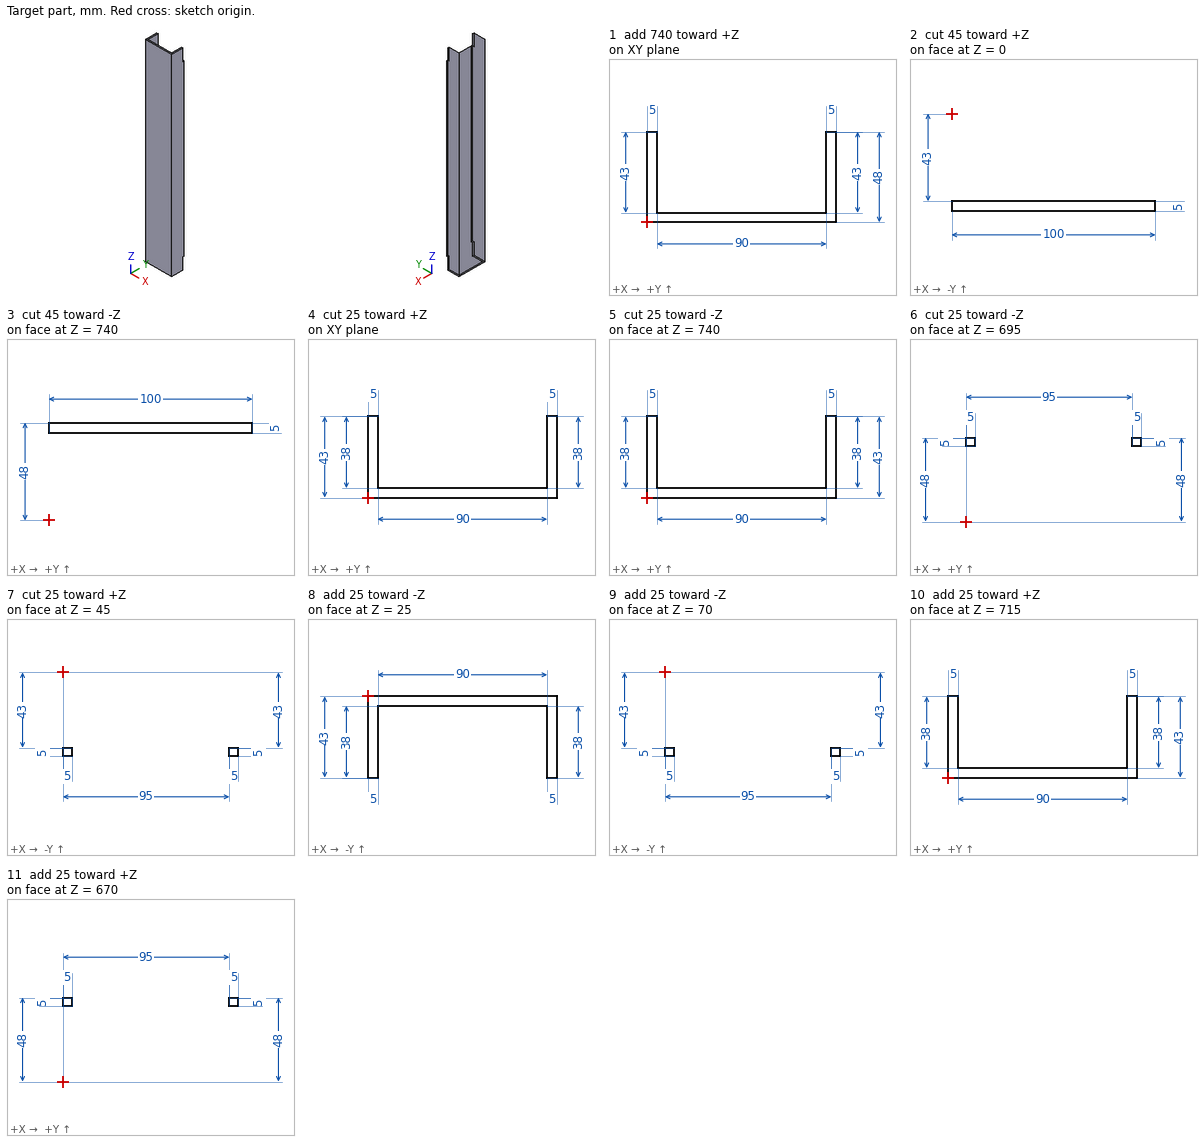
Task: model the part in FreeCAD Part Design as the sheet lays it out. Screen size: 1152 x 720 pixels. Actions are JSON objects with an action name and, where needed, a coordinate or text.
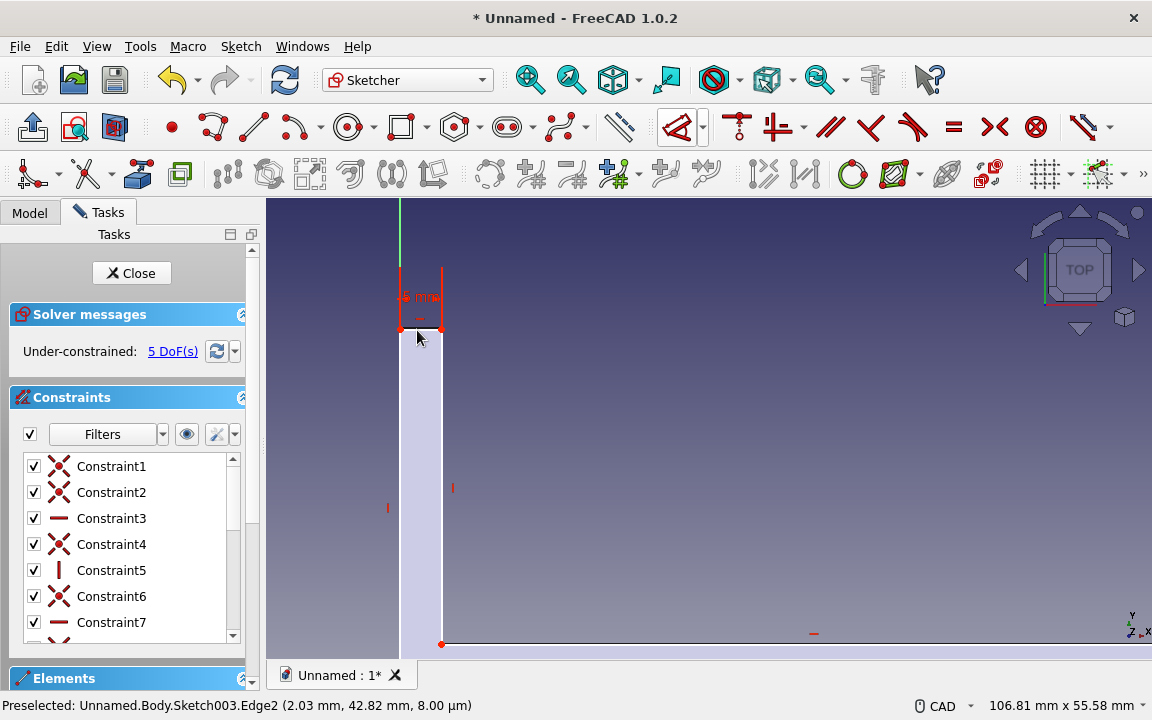
{"action": "scroll", "coordinate": [428, 333], "scroll_direction": "down", "scroll_amount": 3}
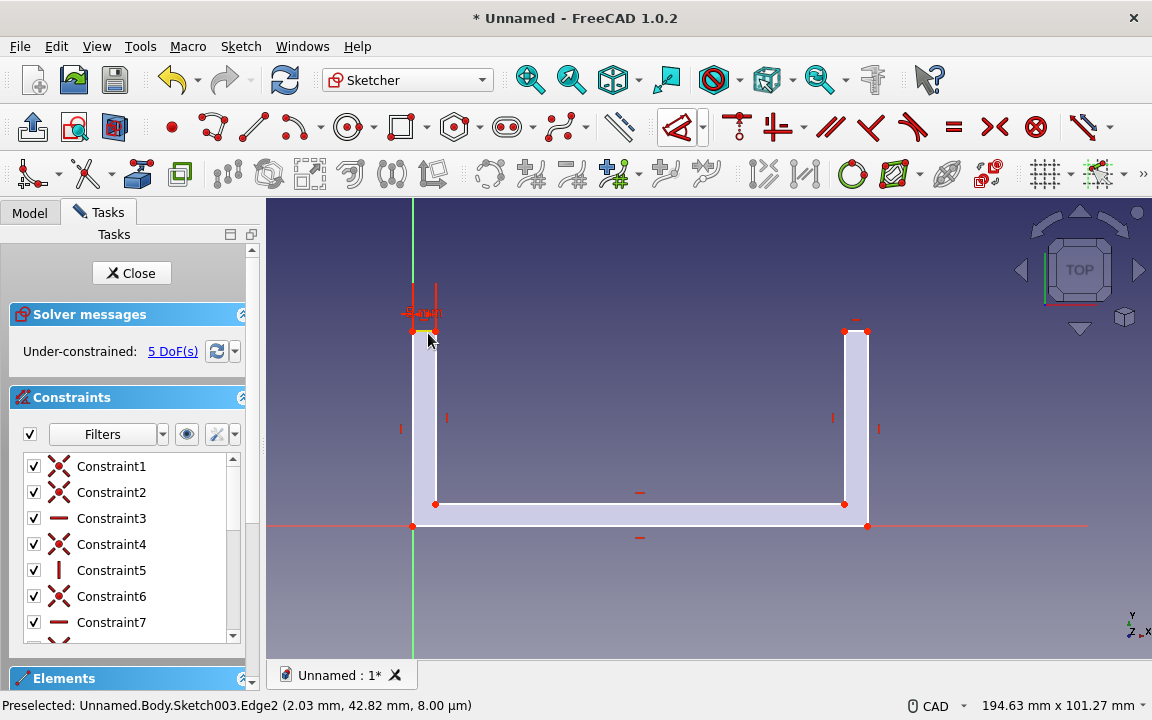
{"action": "scroll", "coordinate": [852, 331], "scroll_direction": "up", "scroll_amount": 4}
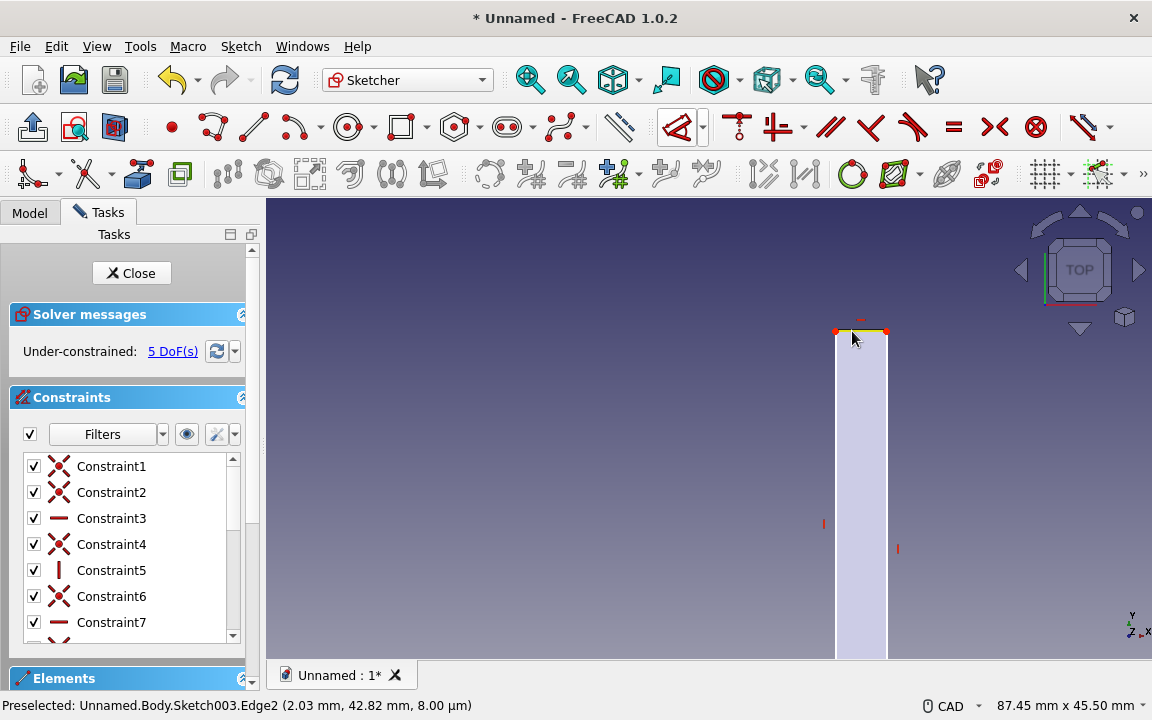
{"action": "left_click", "coordinate": [851, 331]}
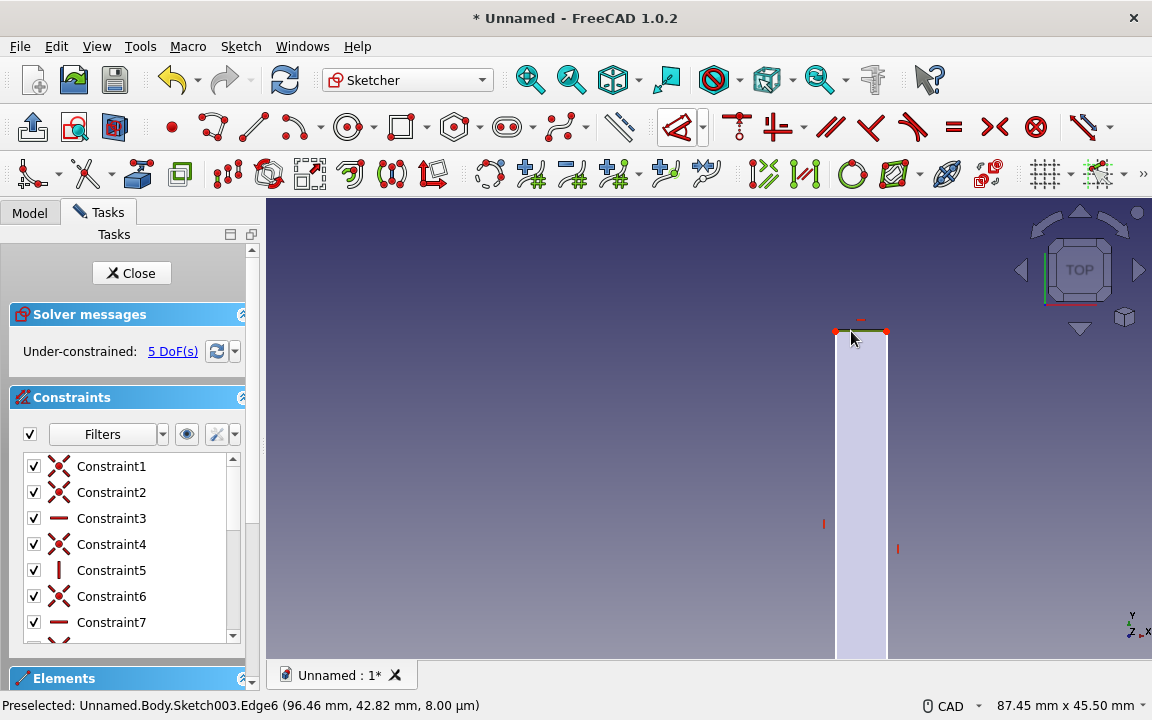
{"action": "left_click", "coordinate": [702, 128]}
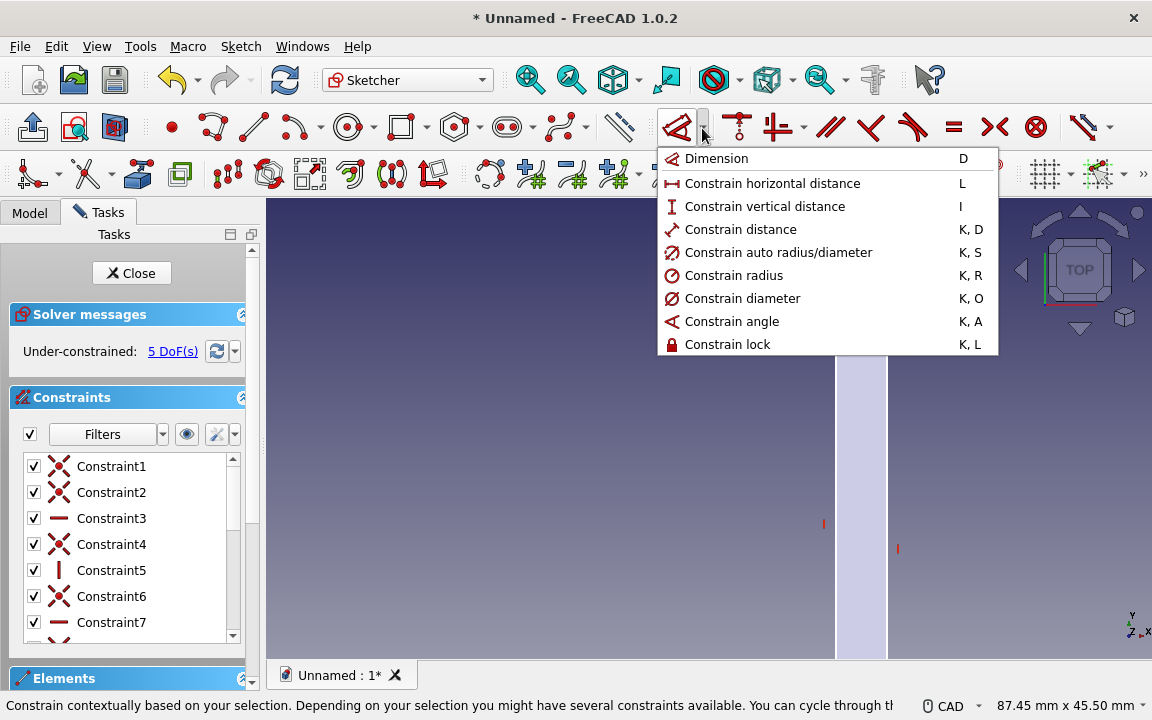
{"action": "left_click", "coordinate": [828, 184]}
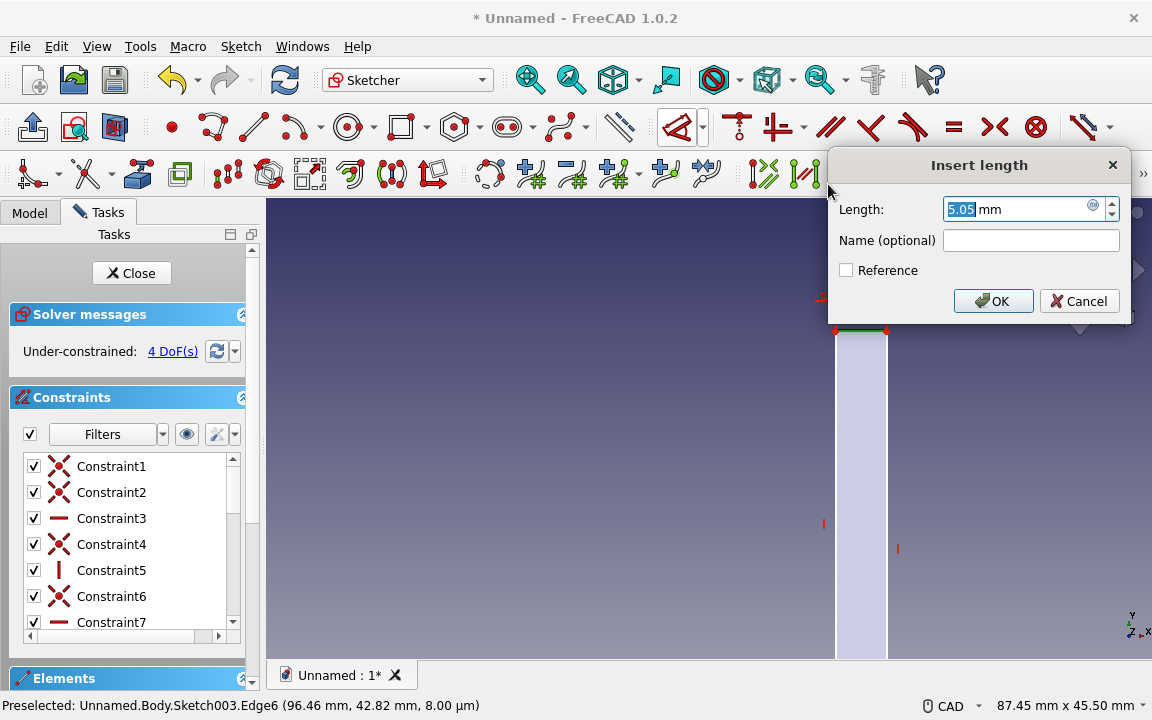
{"action": "type", "text": "5"}
{"action": "key", "text": "Return"}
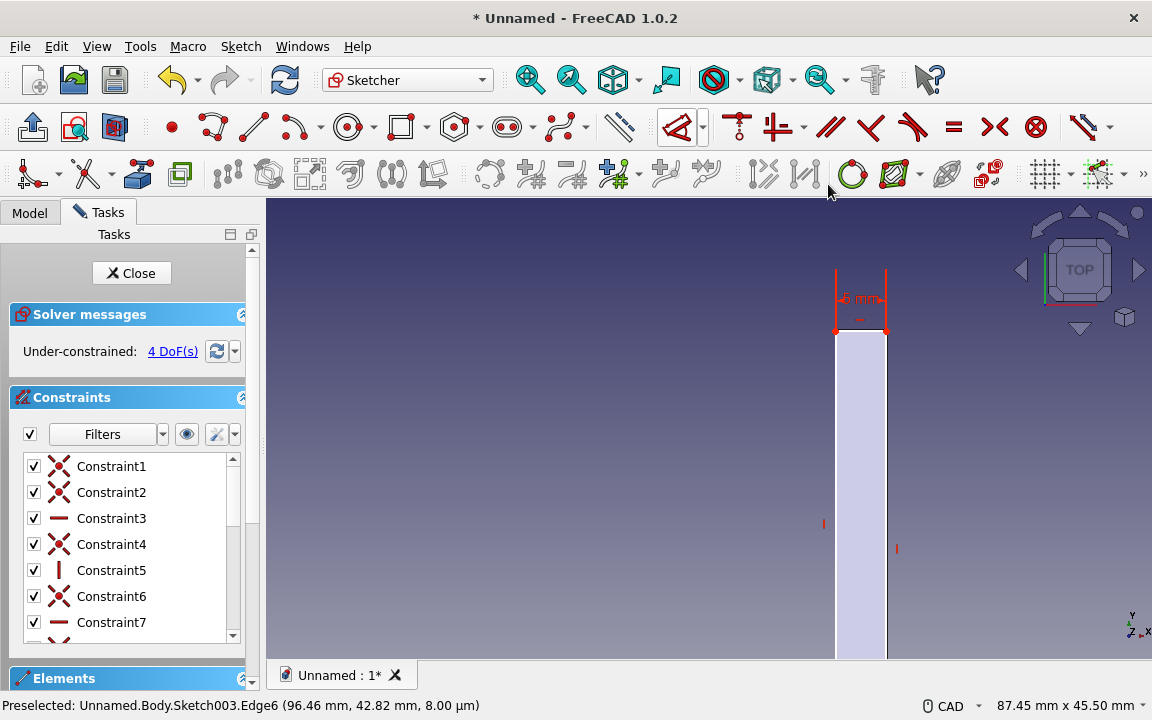
{"action": "scroll", "coordinate": [853, 331], "scroll_direction": "down", "scroll_amount": 4}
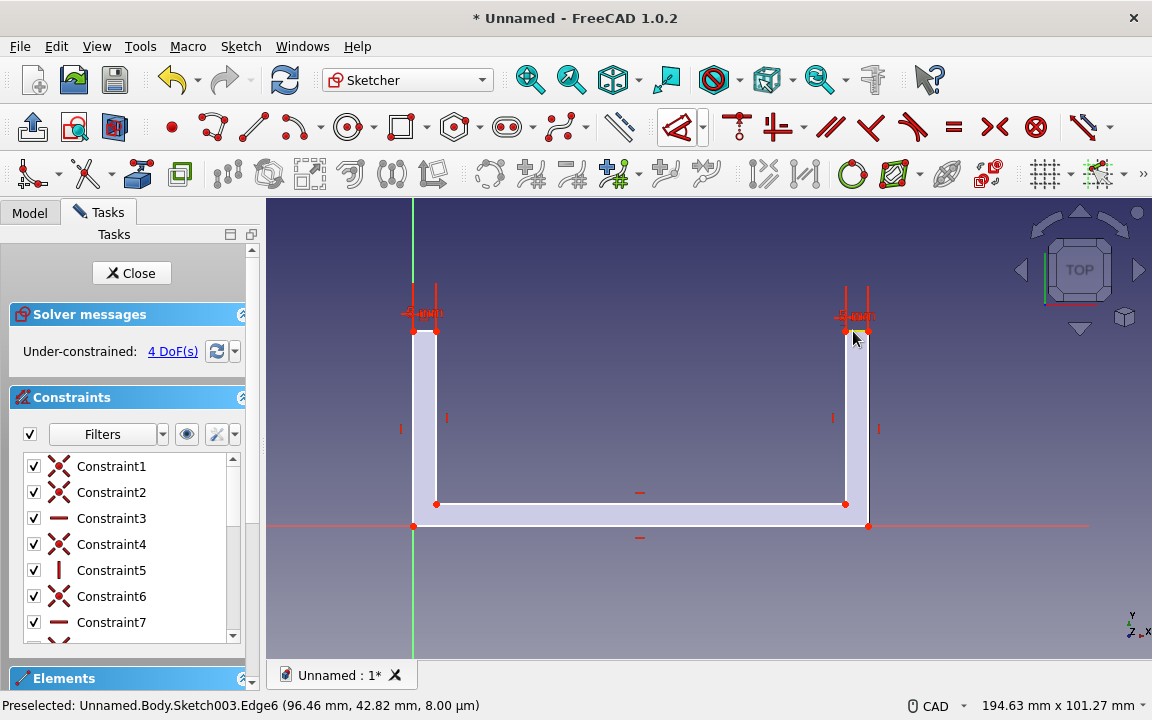
{"action": "left_click", "coordinate": [413, 468]}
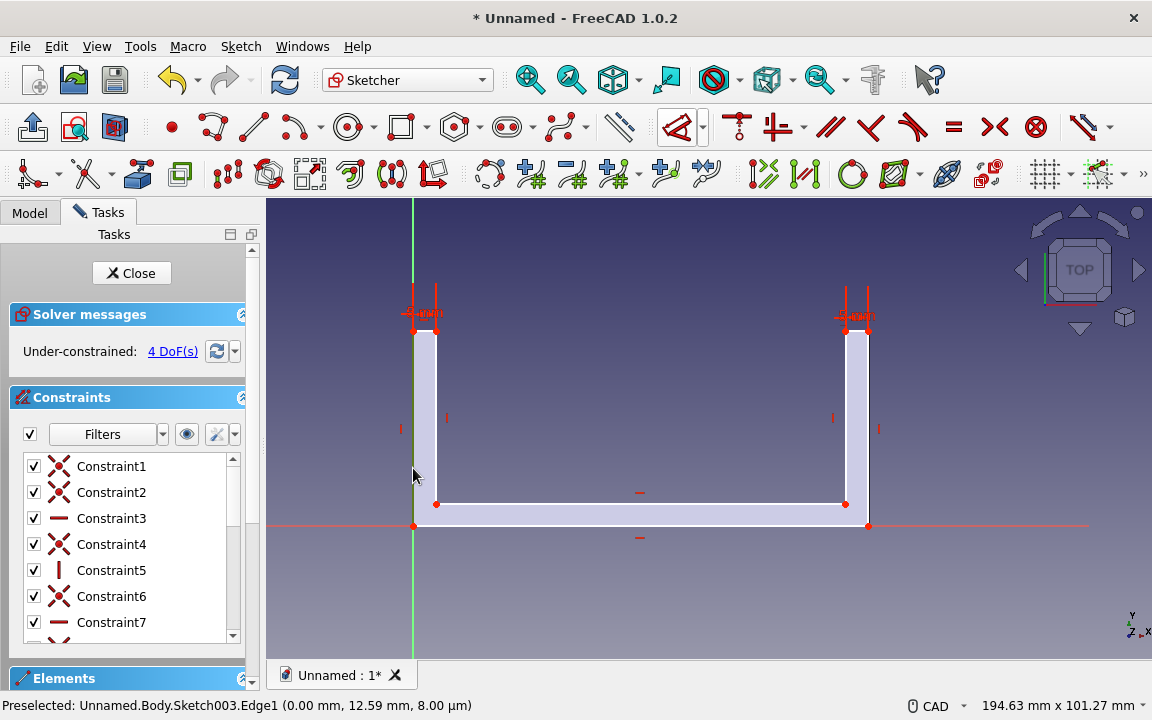
{"action": "left_click", "coordinate": [702, 128]}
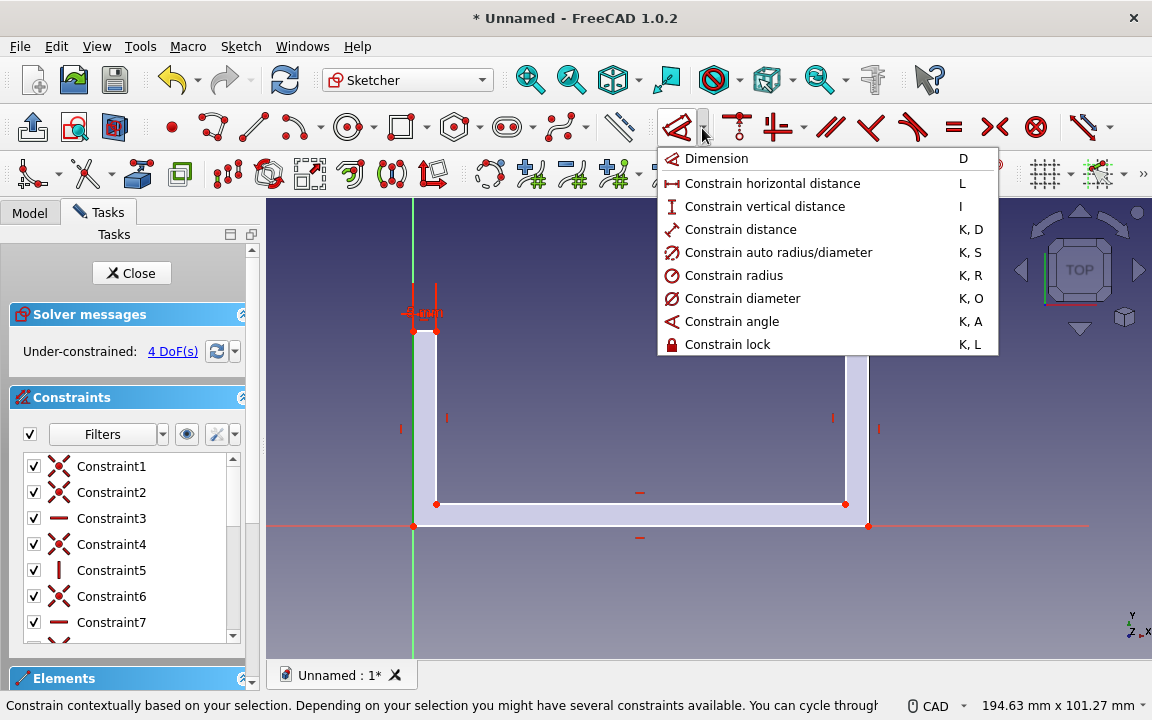
{"action": "left_click", "coordinate": [828, 206]}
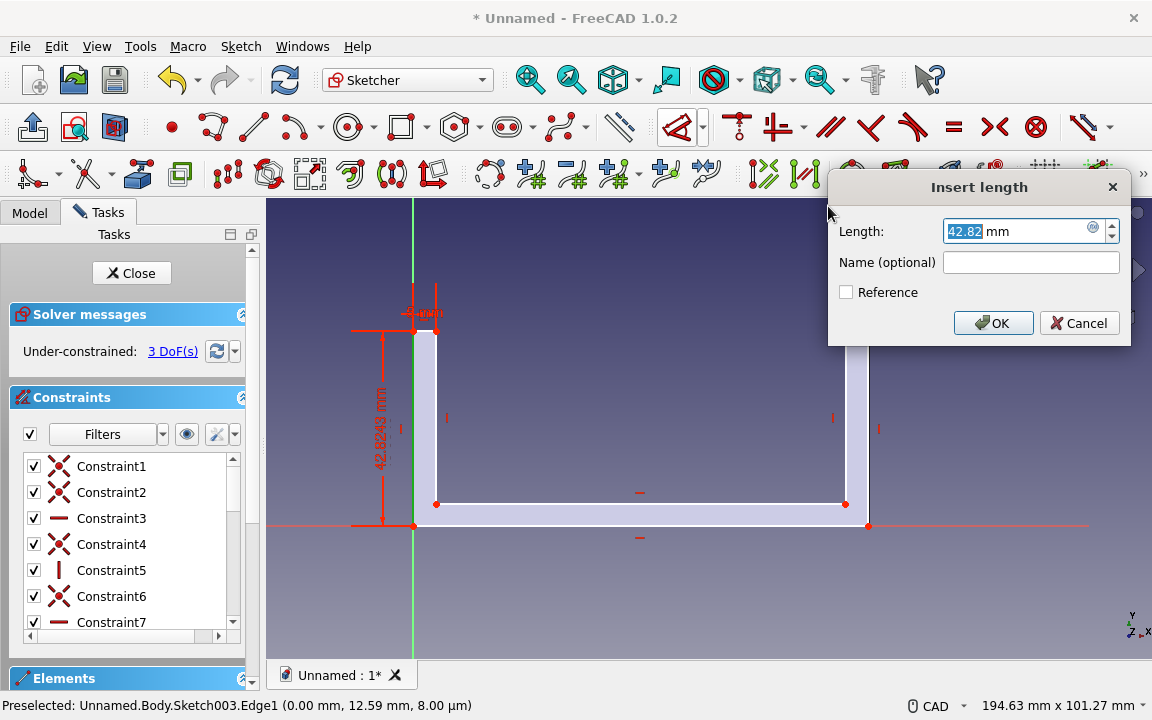
{"action": "type", "text": "43"}
{"action": "key", "text": "Return"}